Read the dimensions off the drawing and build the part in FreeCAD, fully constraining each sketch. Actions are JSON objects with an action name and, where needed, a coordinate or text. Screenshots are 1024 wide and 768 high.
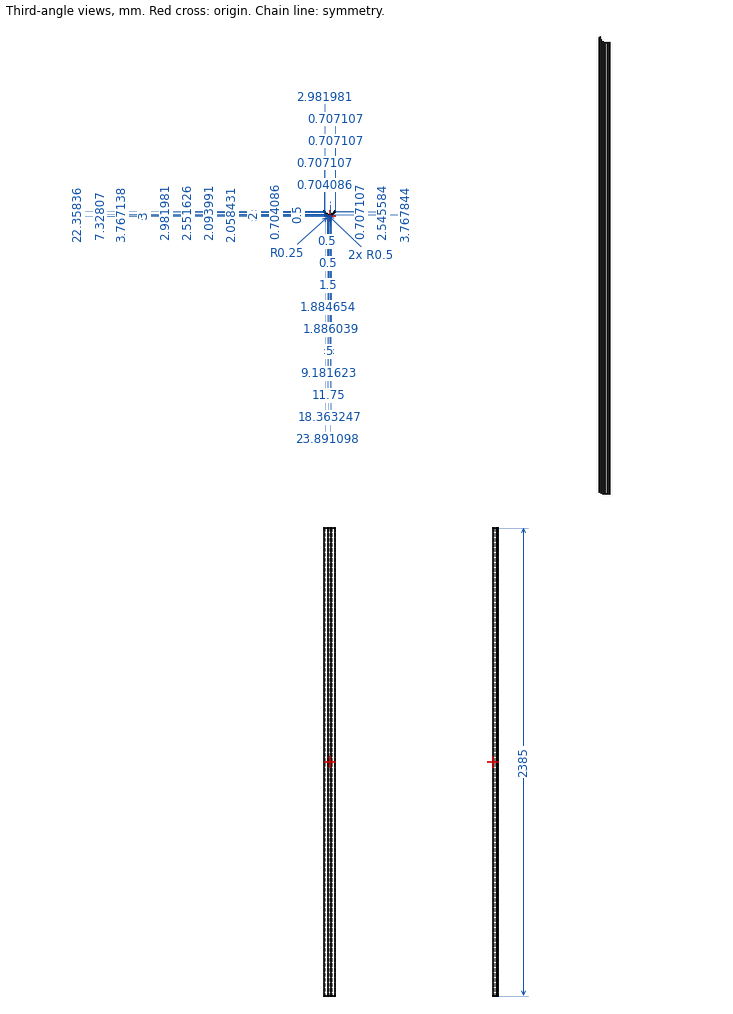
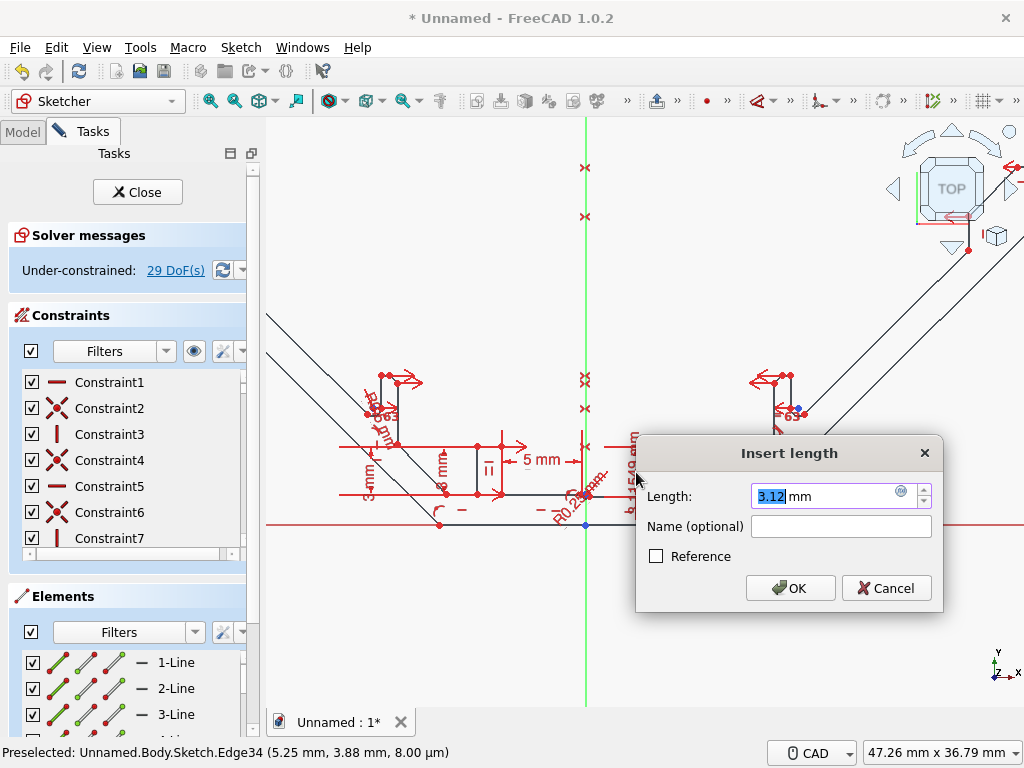
{"action": "type", "text": "3"}
{"action": "key", "text": "Return"}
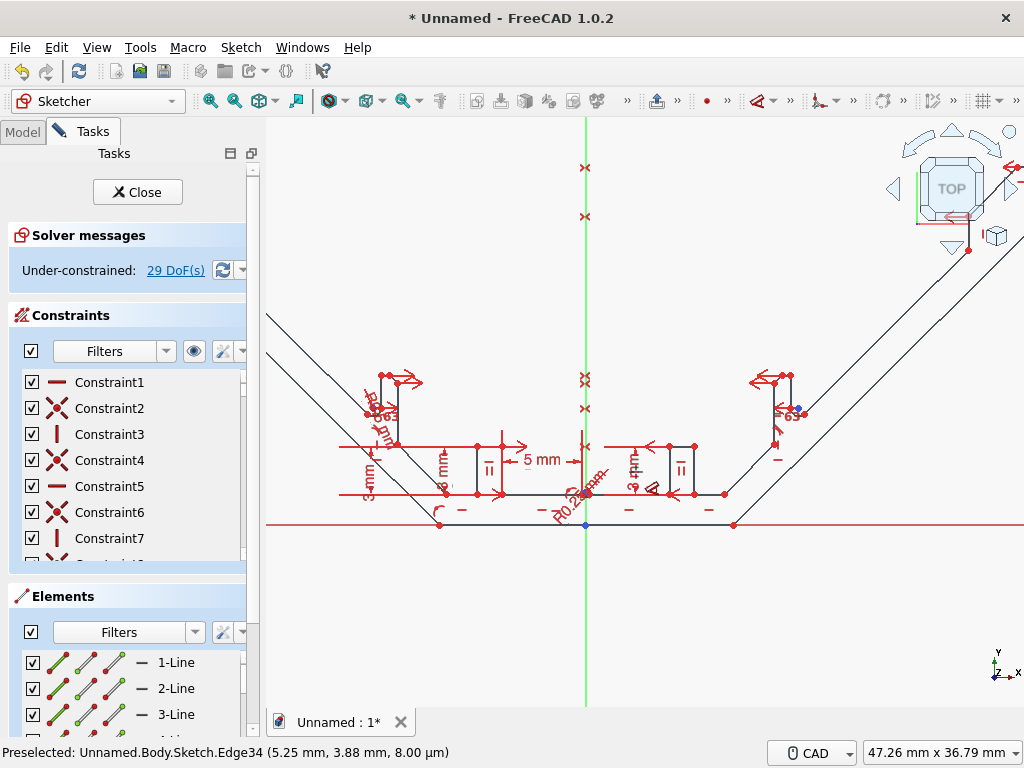
{"action": "scroll", "coordinate": [582, 495], "scroll_direction": "up", "scroll_amount": 6}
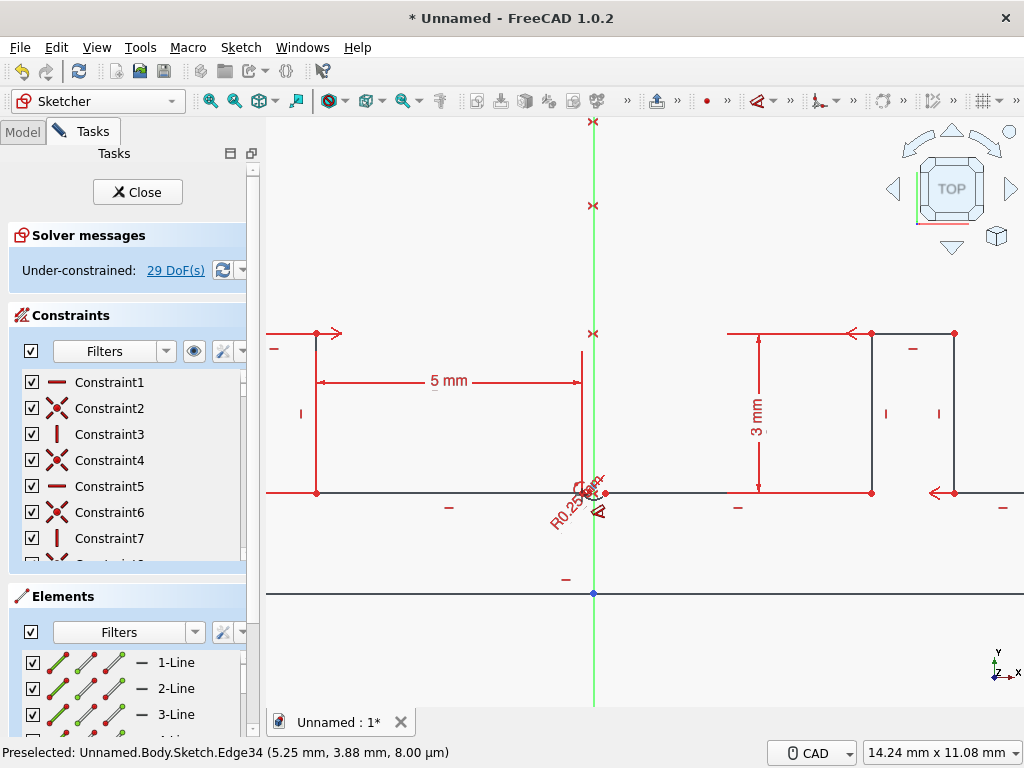
{"action": "left_click", "coordinate": [582, 493]}
{"action": "left_click", "coordinate": [548, 544]}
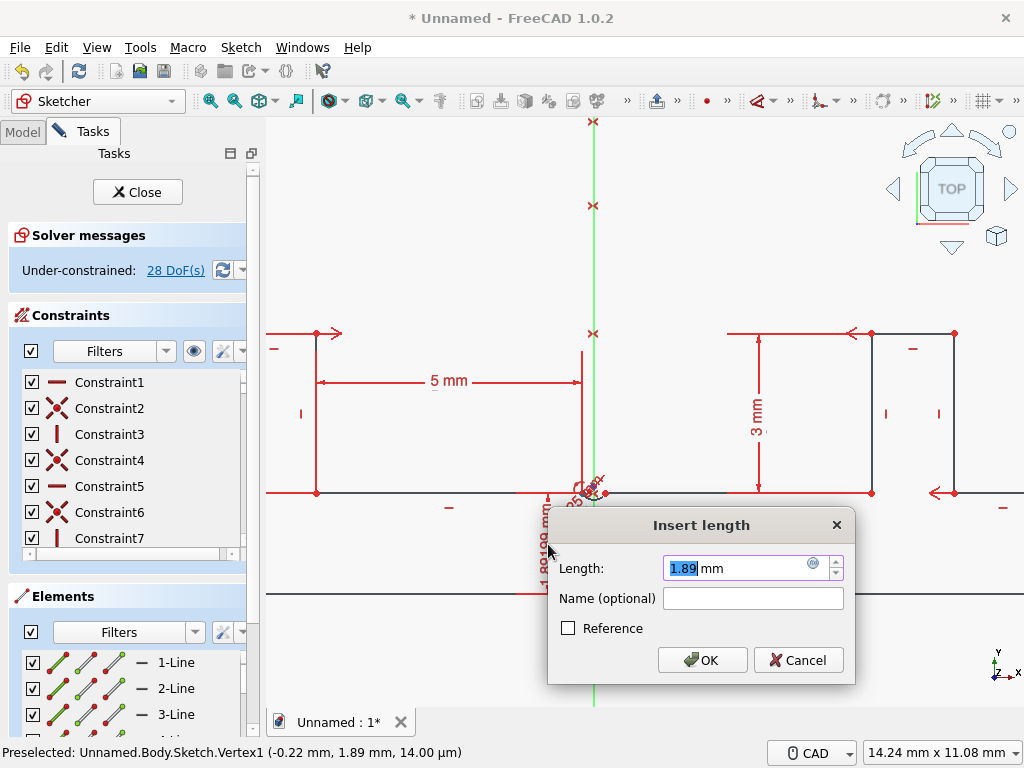
{"action": "type", "text": "2"}
{"action": "key", "text": "Return"}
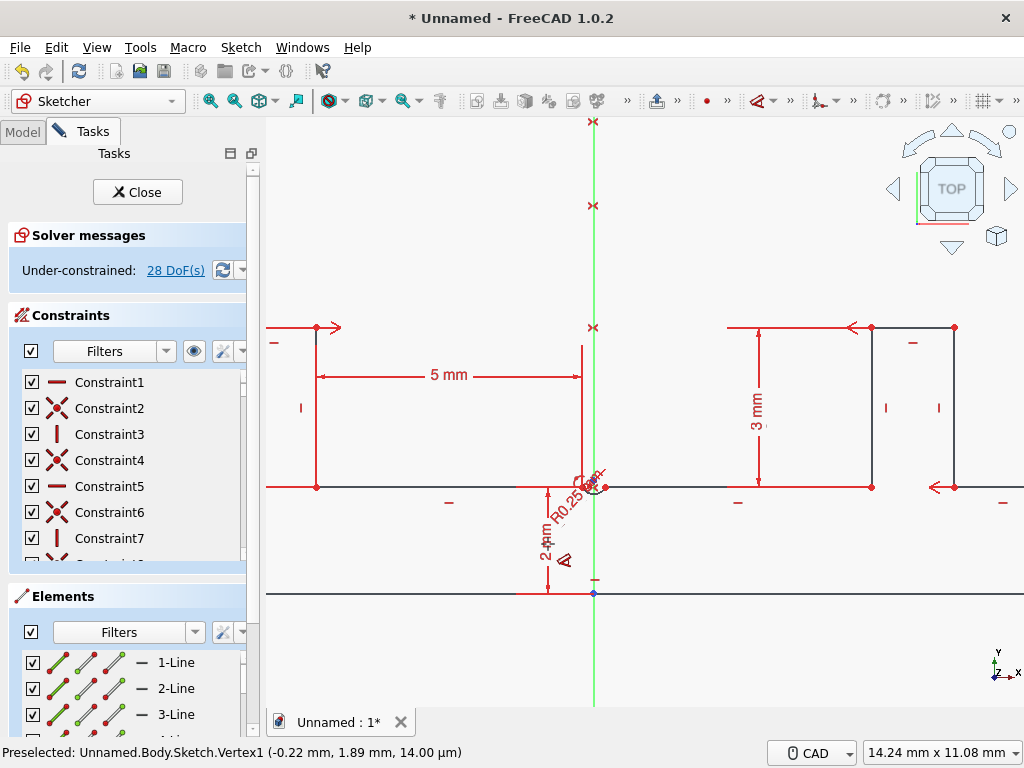
{"action": "left_click", "coordinate": [594, 481]}
{"action": "left_click", "coordinate": [560, 577]}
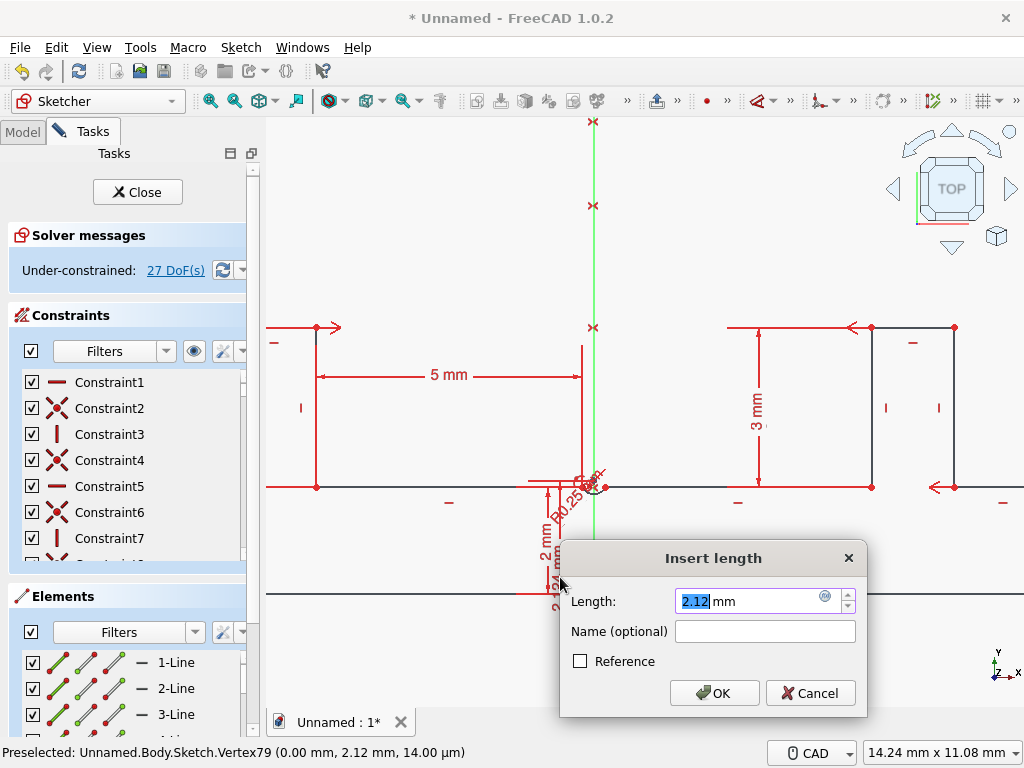
{"action": "type", "text": "2"}
{"action": "key", "text": "Return"}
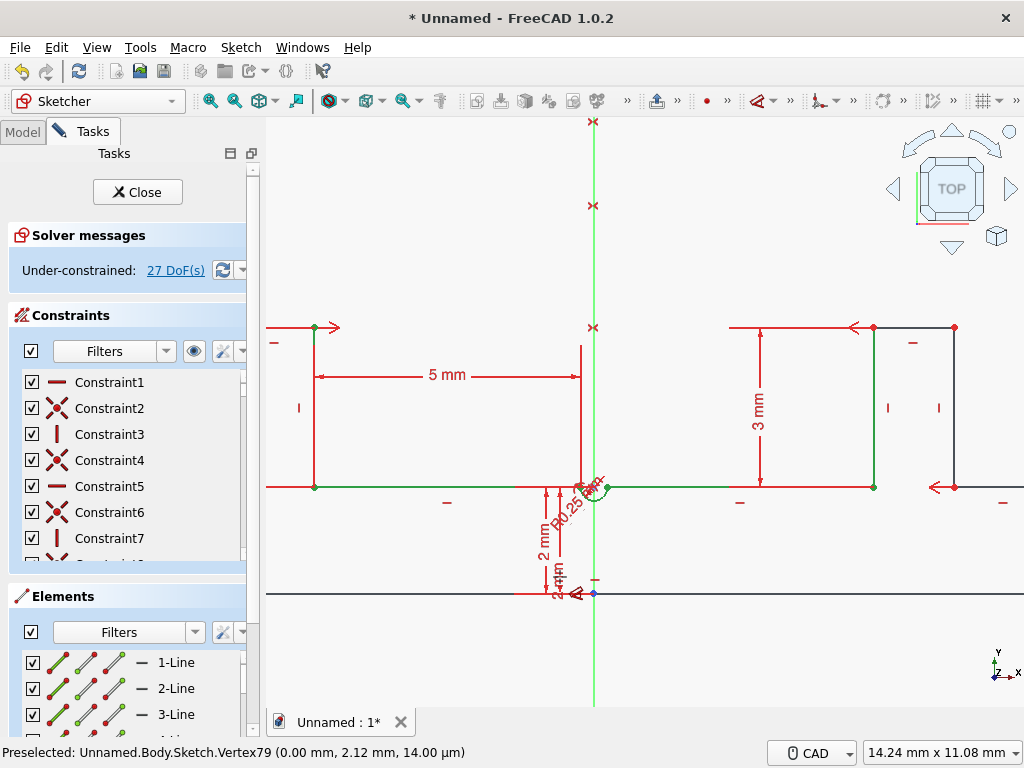
{"action": "left_click", "coordinate": [298, 328]}
{"action": "left_click", "coordinate": [300, 362]}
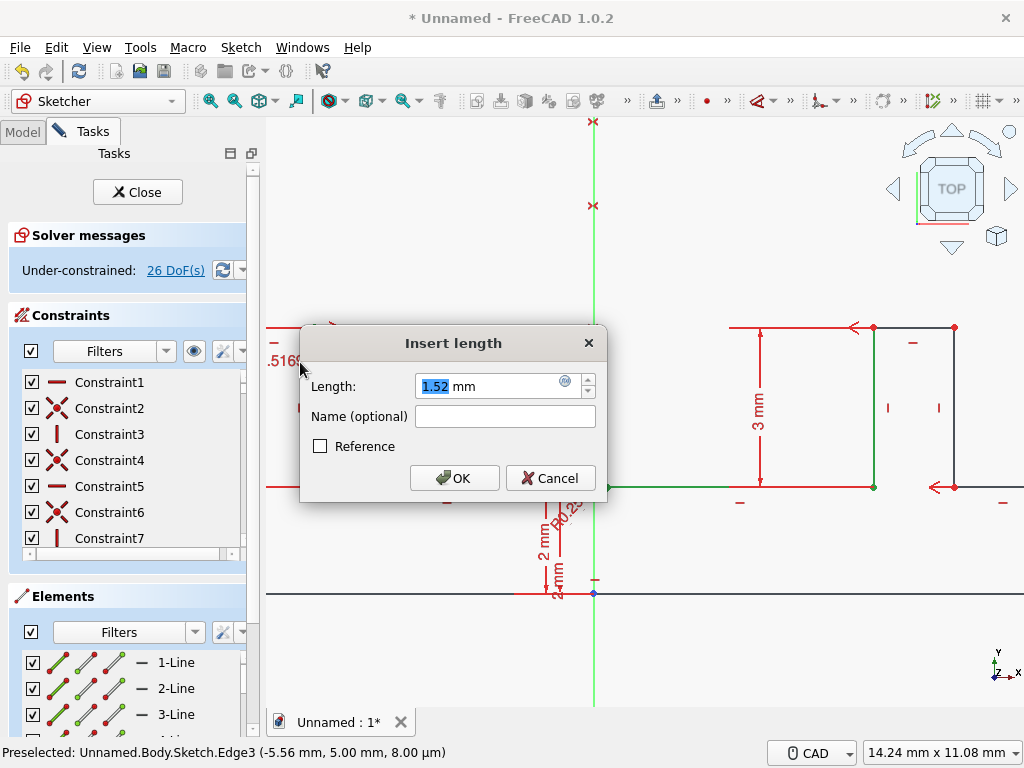
{"action": "type", "text": "1.5"}
{"action": "key", "text": "Return"}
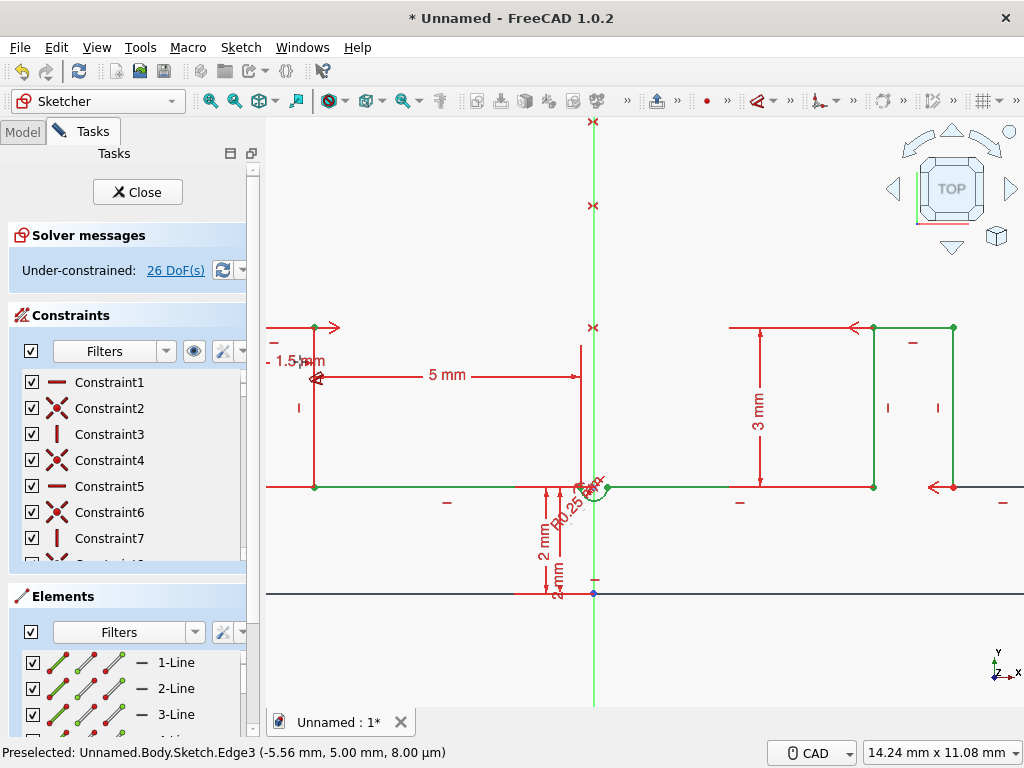
{"action": "scroll", "coordinate": [574, 477], "scroll_direction": "down", "scroll_amount": 10}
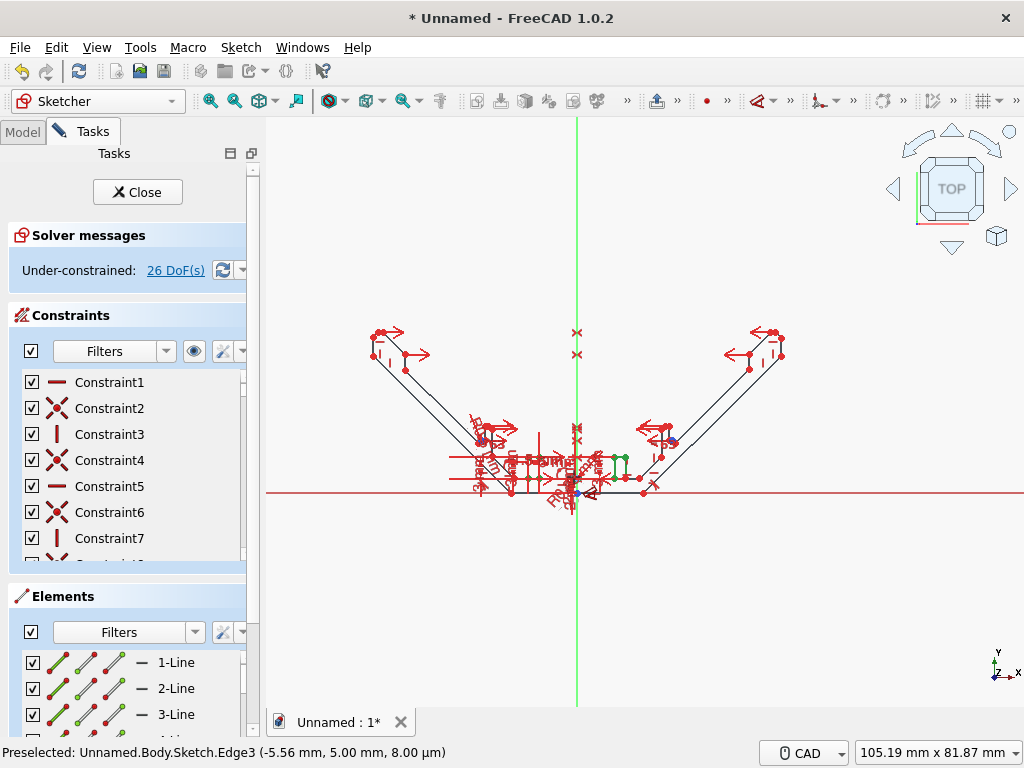
{"action": "scroll", "coordinate": [487, 426], "scroll_direction": "up", "scroll_amount": 12}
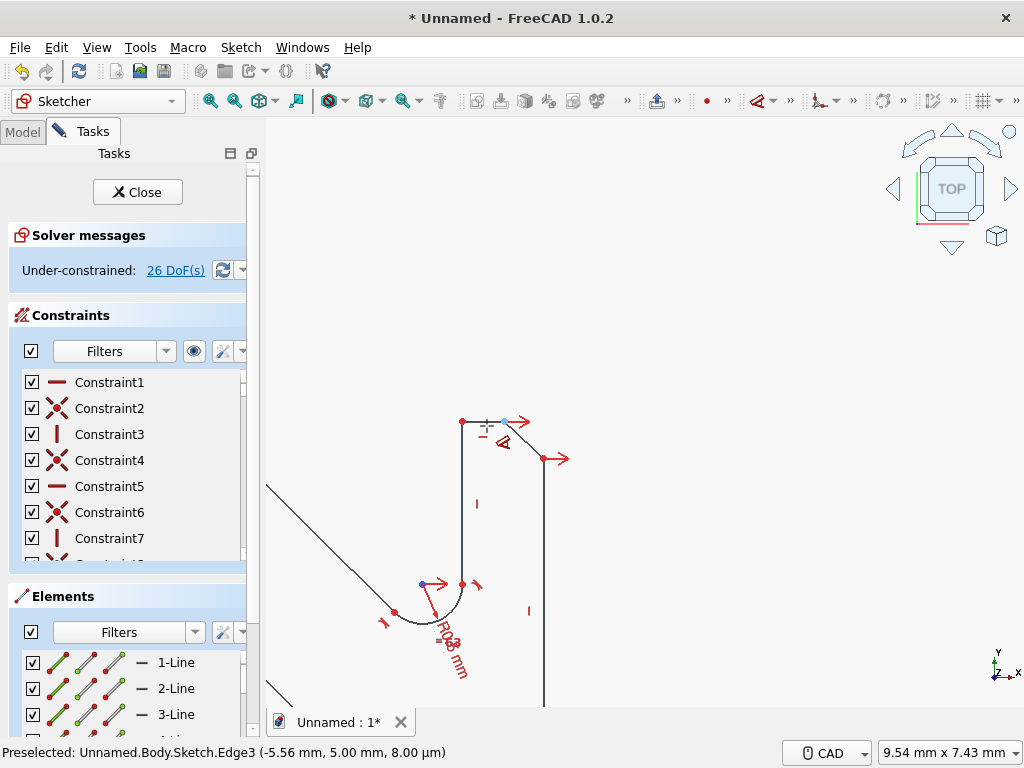
{"action": "left_click", "coordinate": [488, 422]}
{"action": "left_click", "coordinate": [484, 456]}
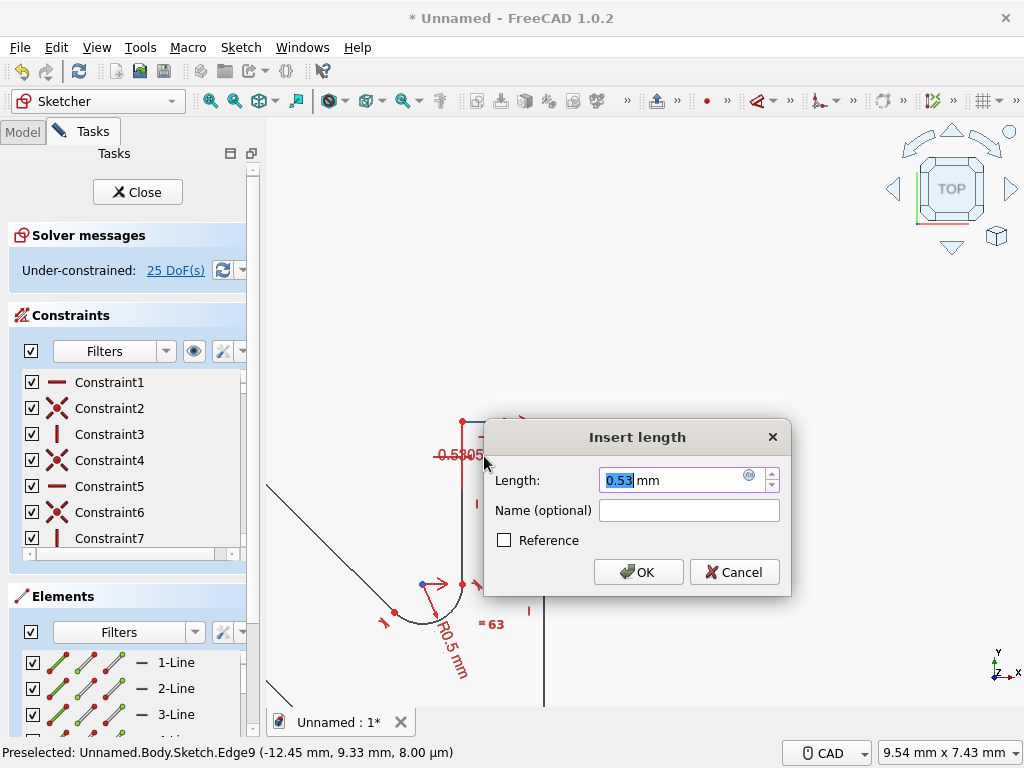
{"action": "type", "text": "0.5"}
{"action": "key", "text": "Return"}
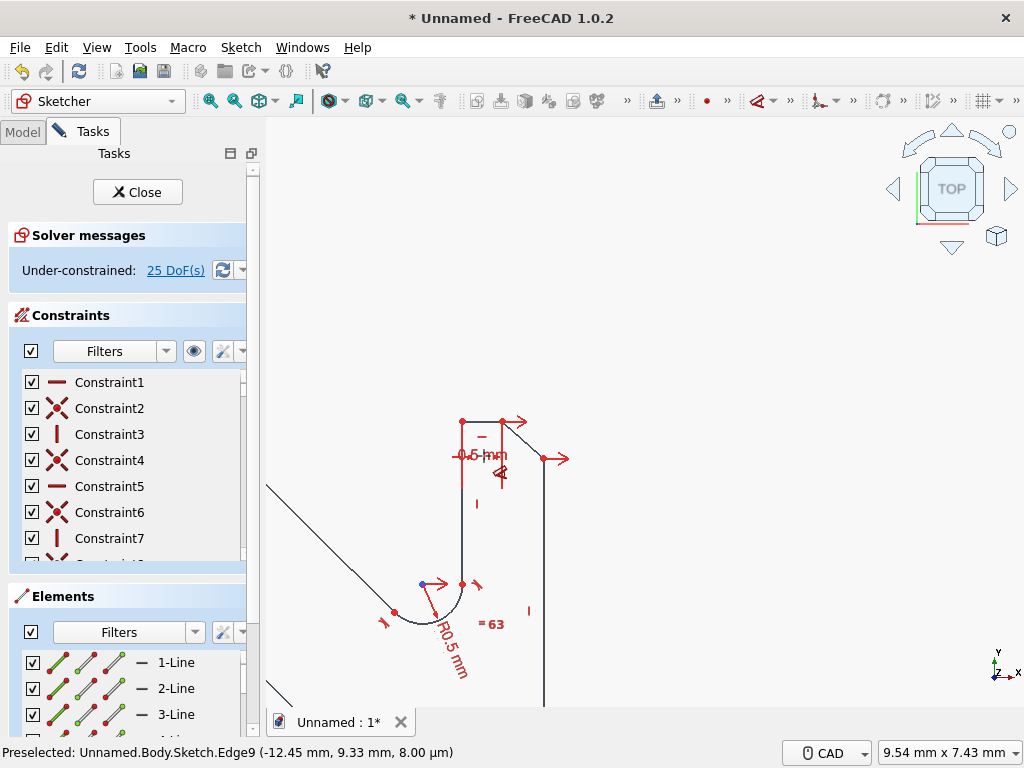
{"action": "left_click", "coordinate": [531, 448]}
{"action": "left_click", "coordinate": [523, 493]}